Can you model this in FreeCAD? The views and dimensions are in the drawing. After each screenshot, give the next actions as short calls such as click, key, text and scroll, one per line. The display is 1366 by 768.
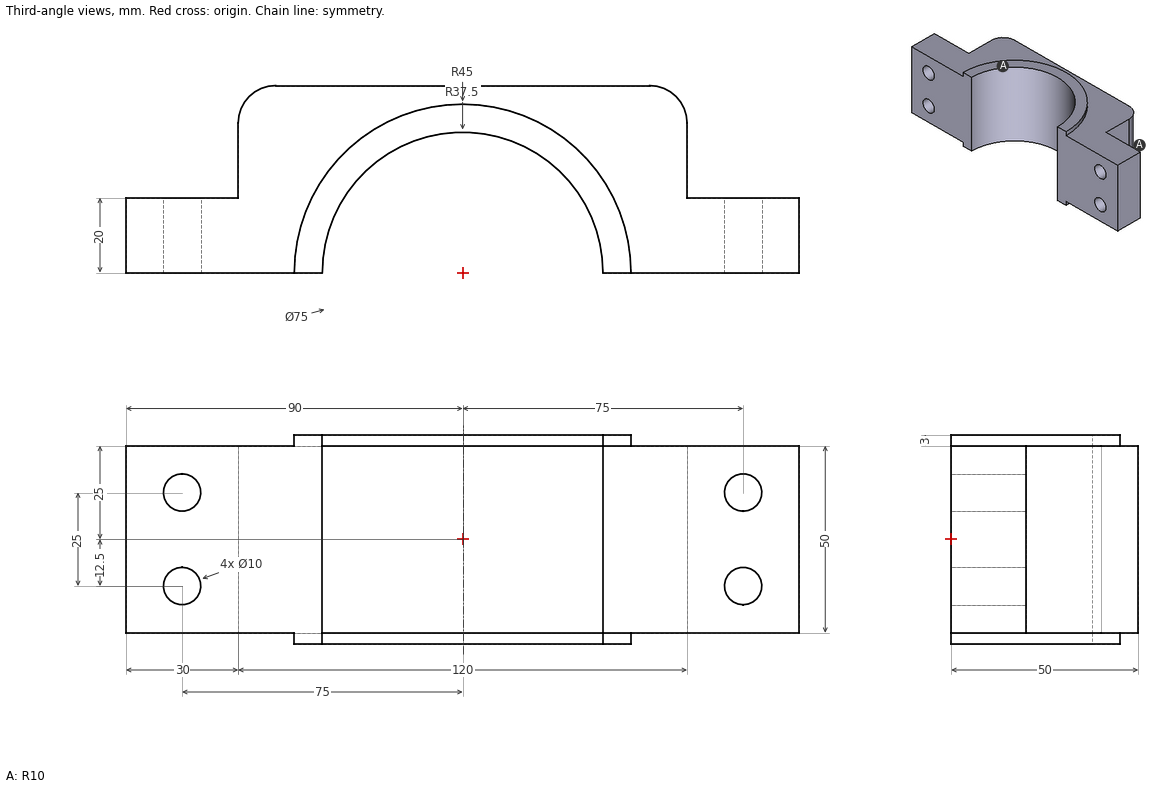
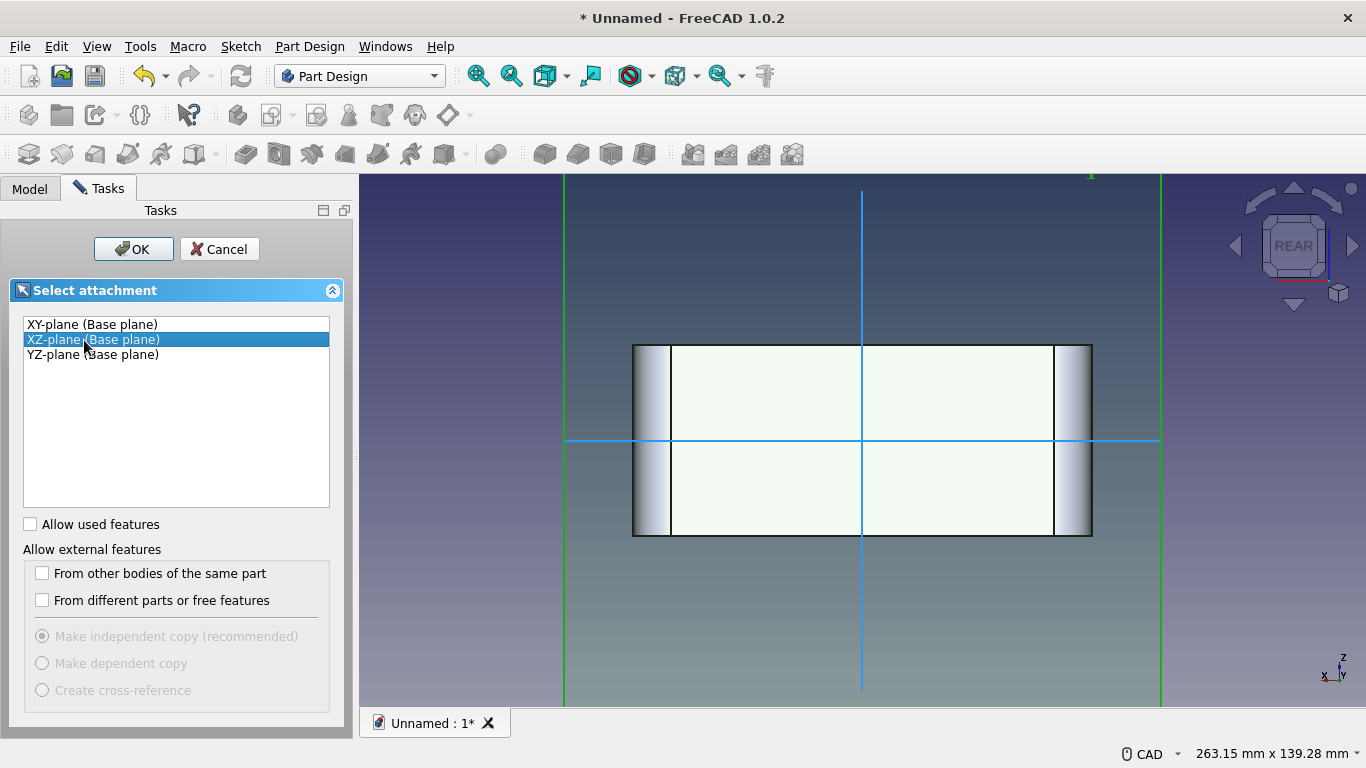
click(134, 249)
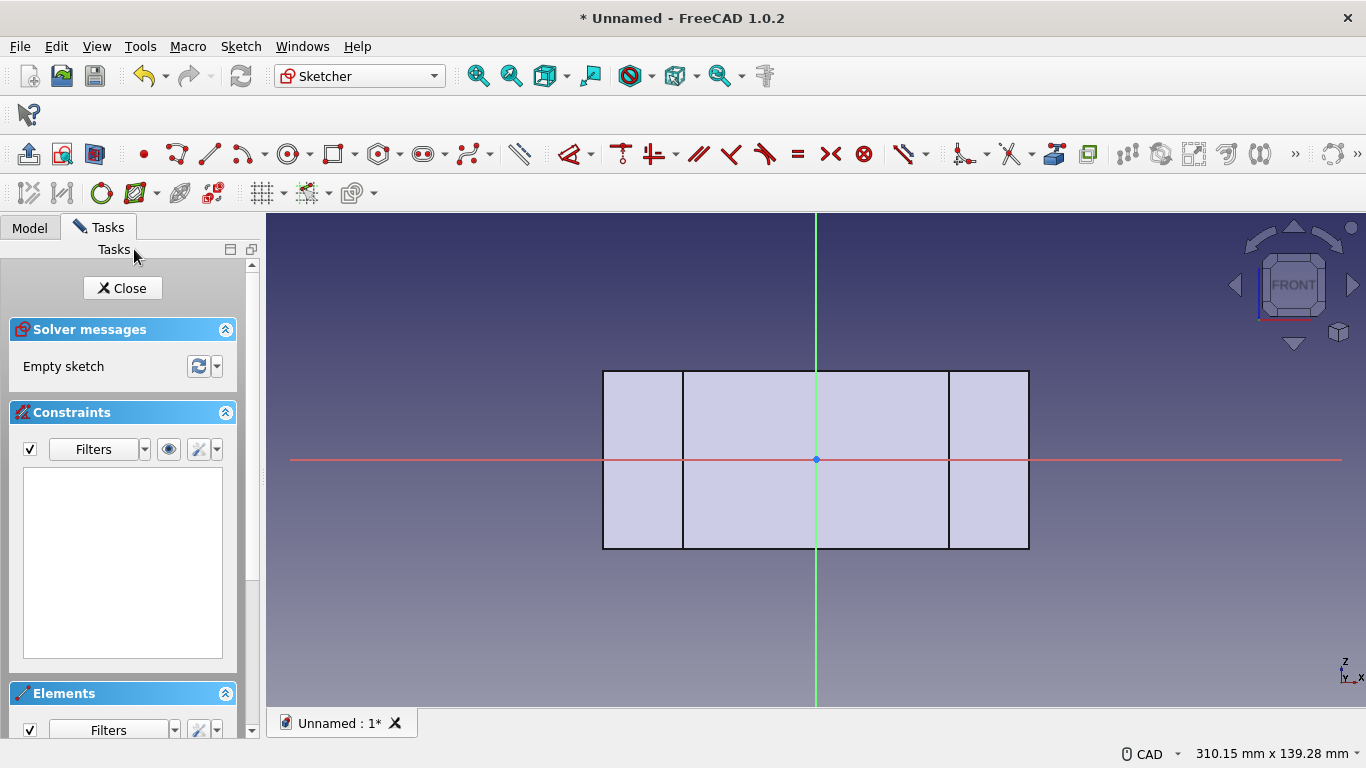
key(g)
key(r)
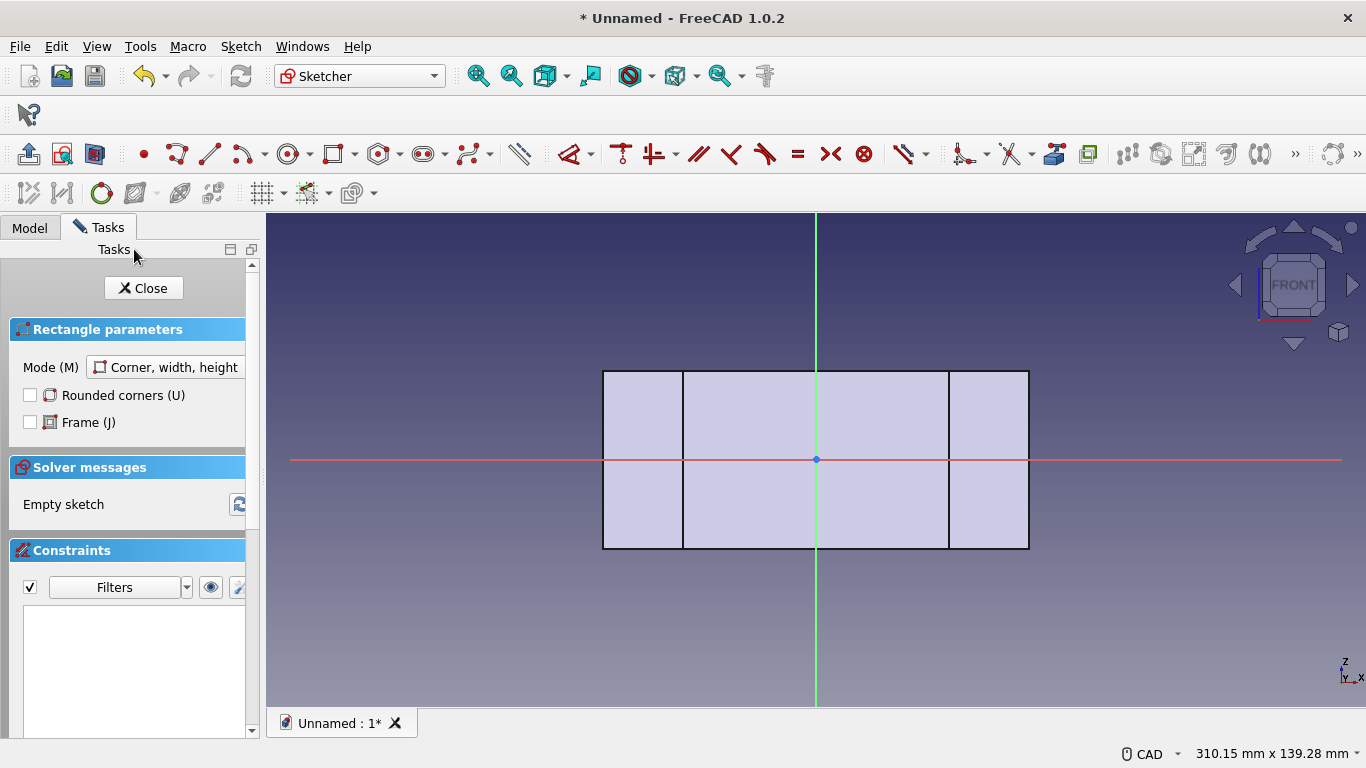
click(497, 371)
click(603, 549)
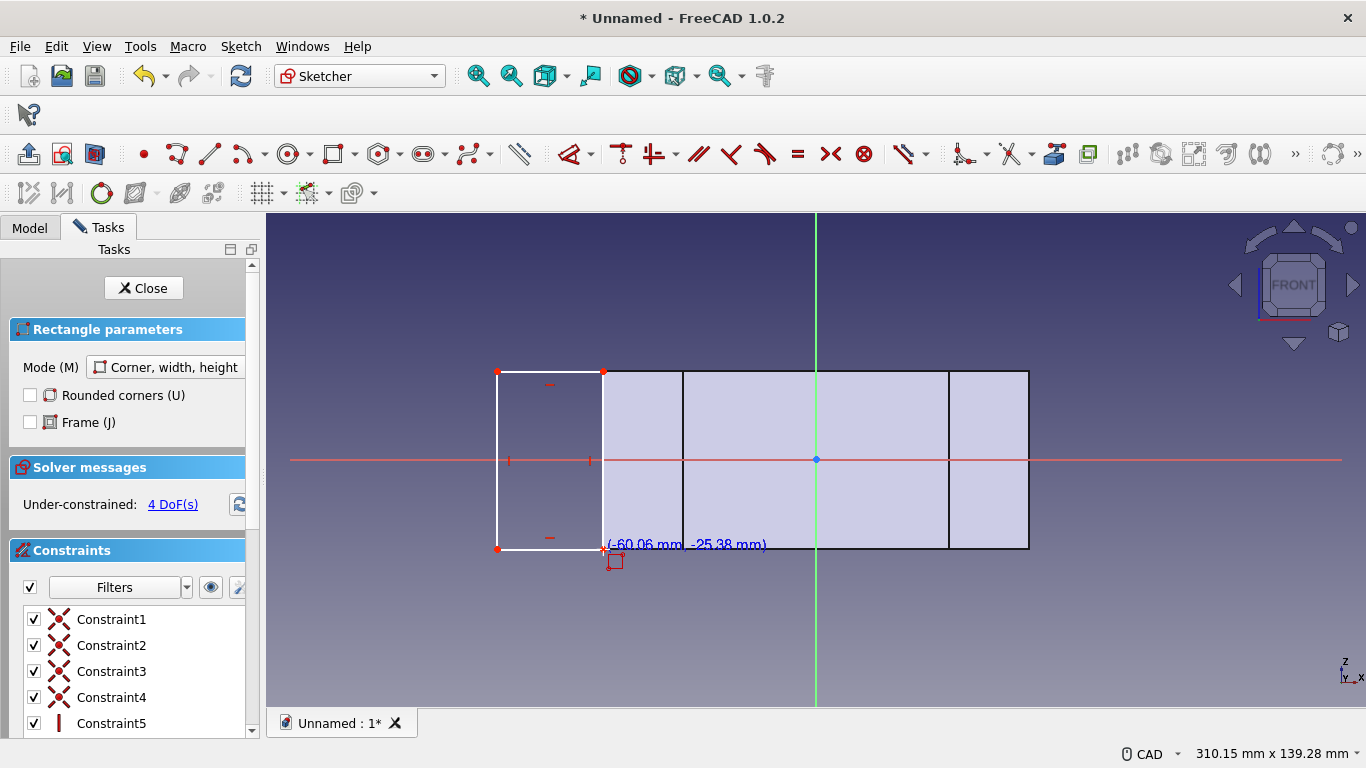
click(1029, 371)
click(1135, 549)
key(Escape)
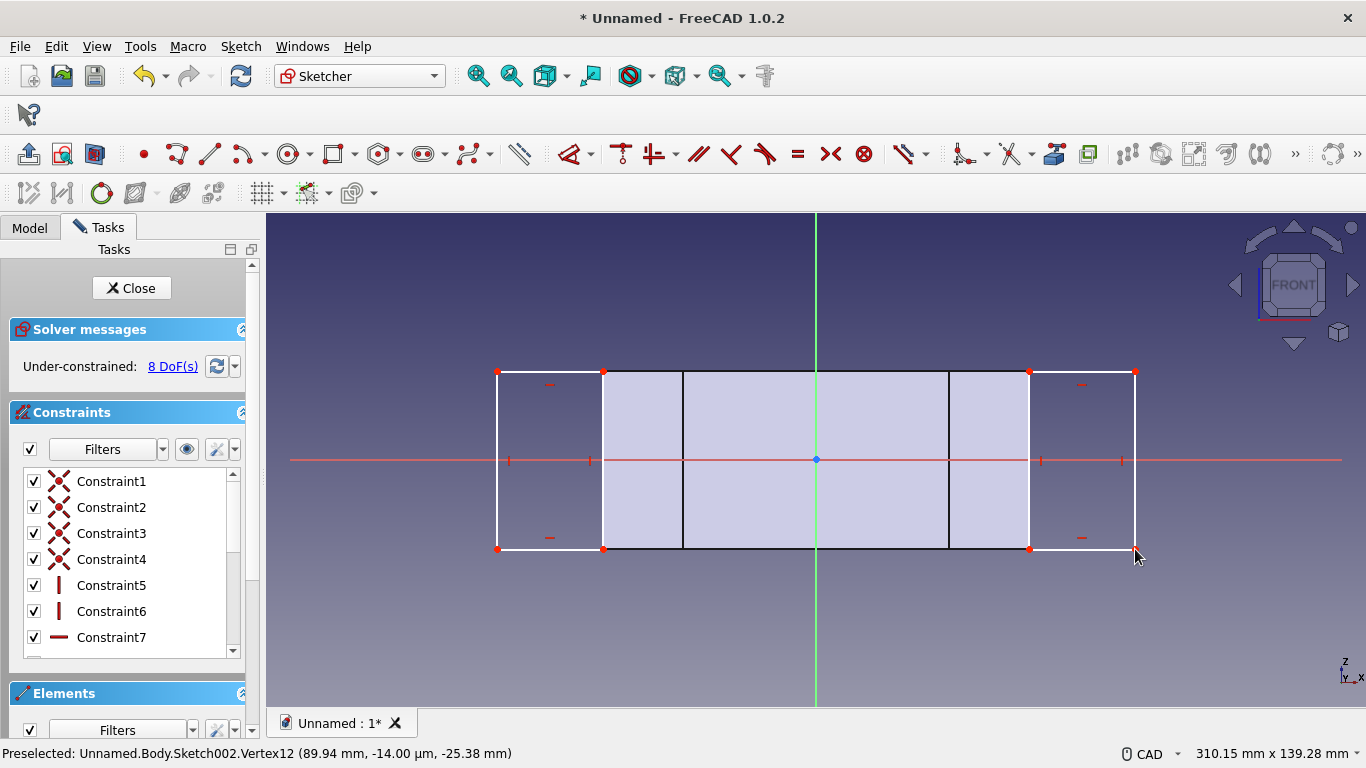
click(603, 372)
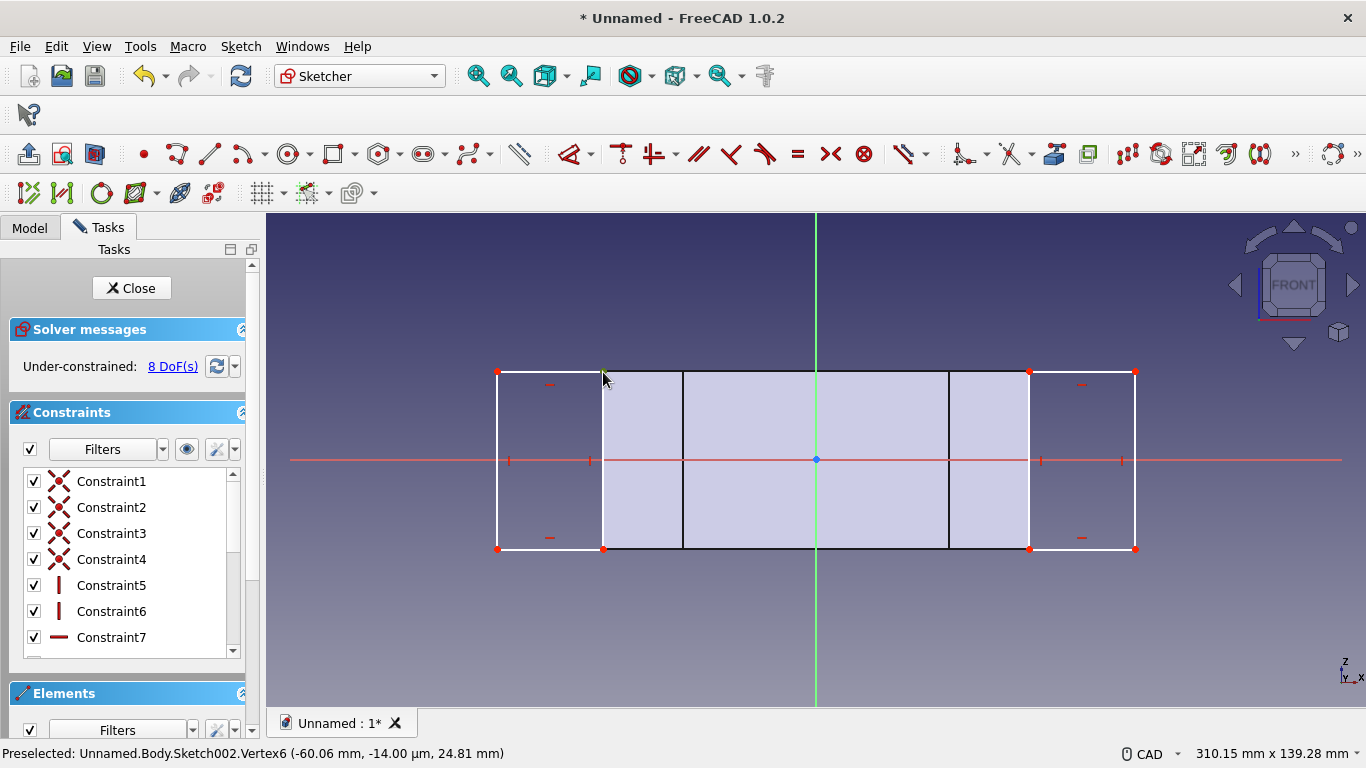
click(1029, 372)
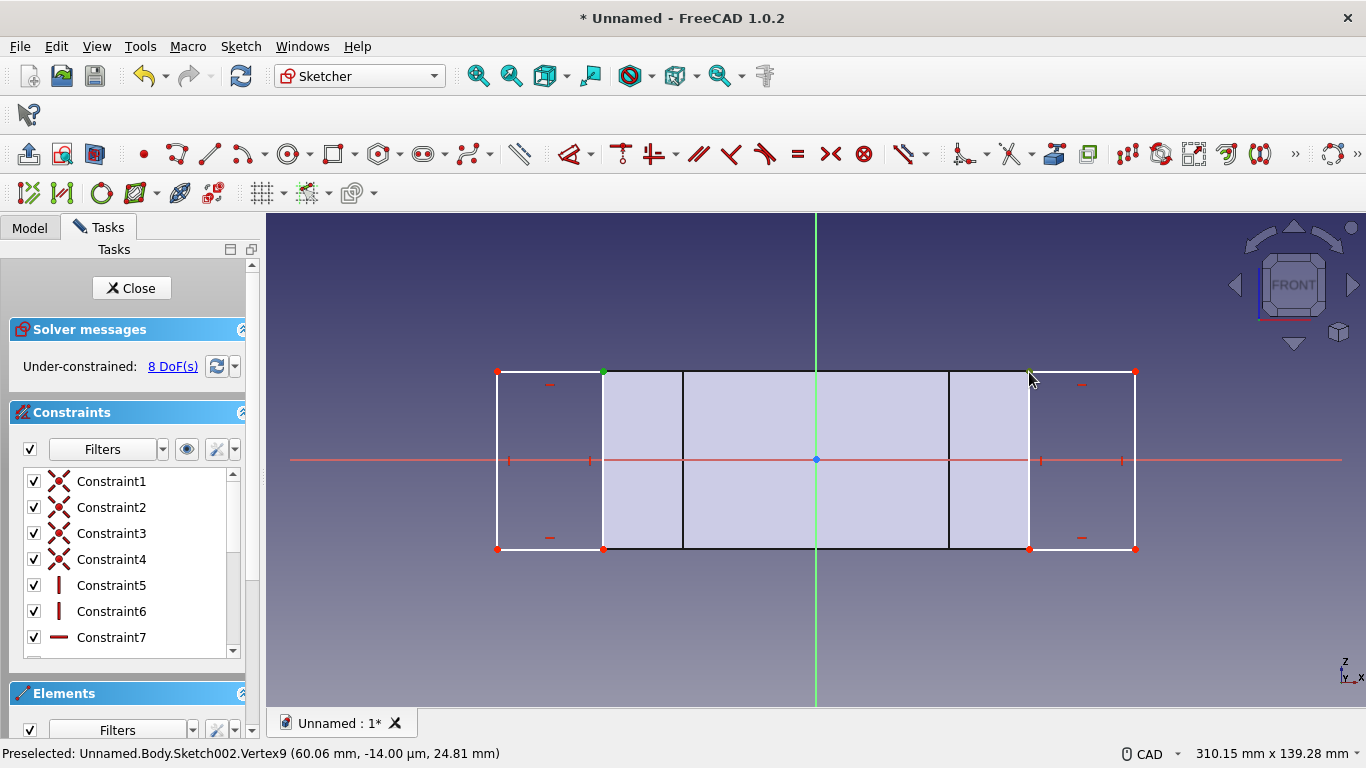
click(816, 648)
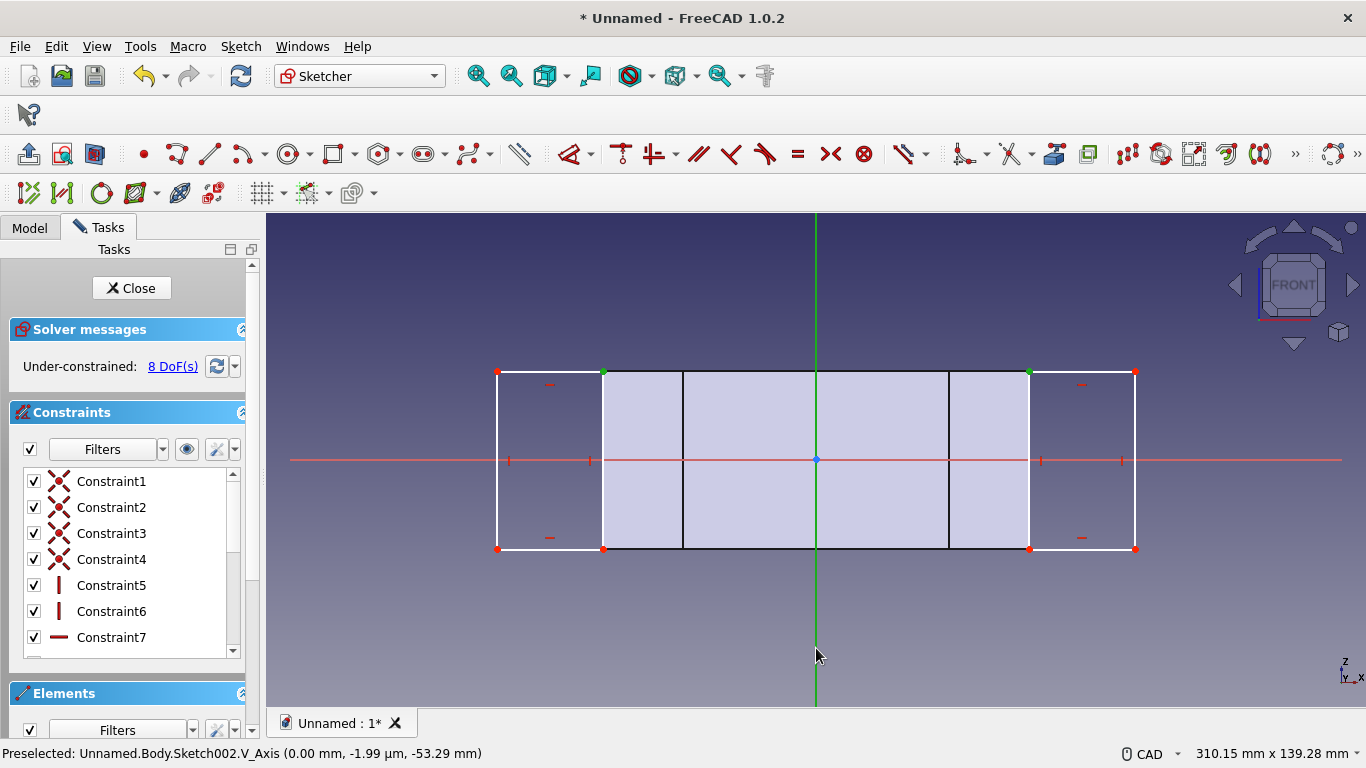
key(s)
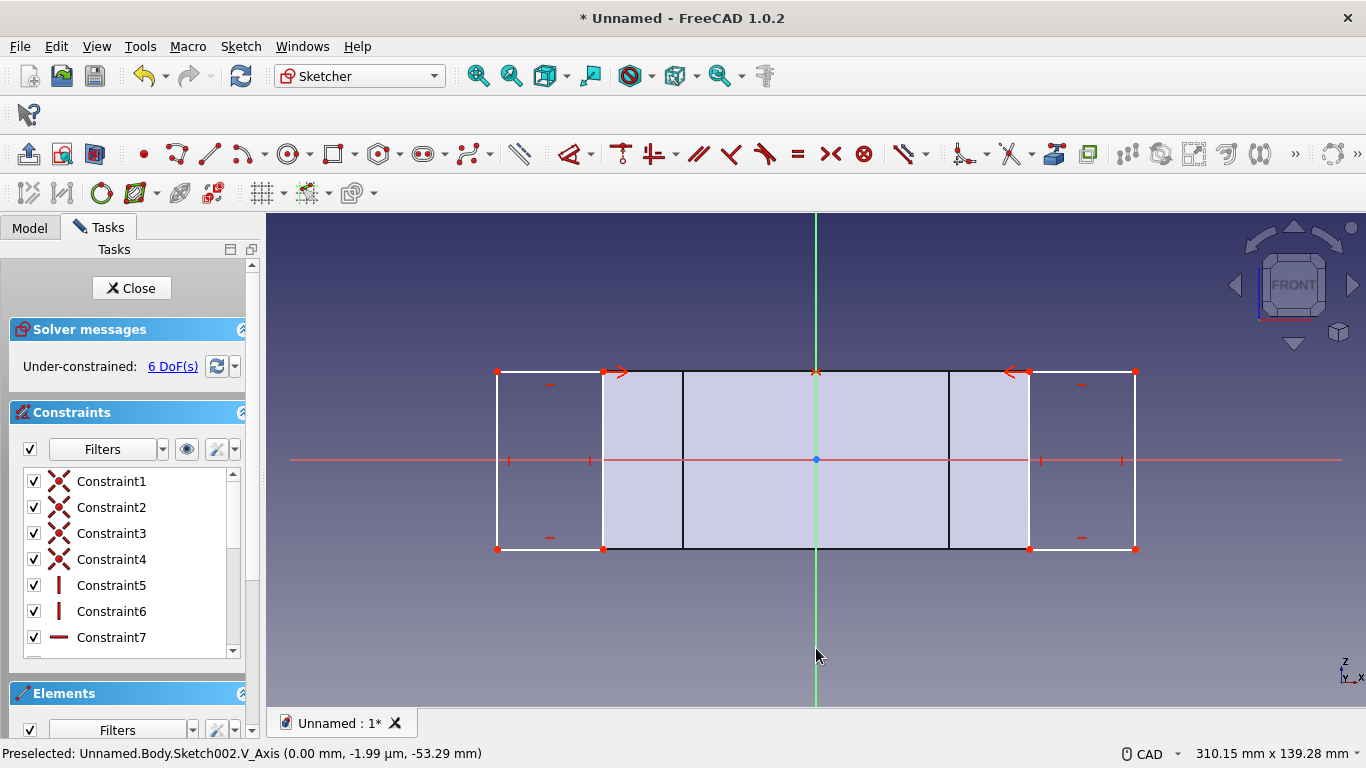
click(497, 550)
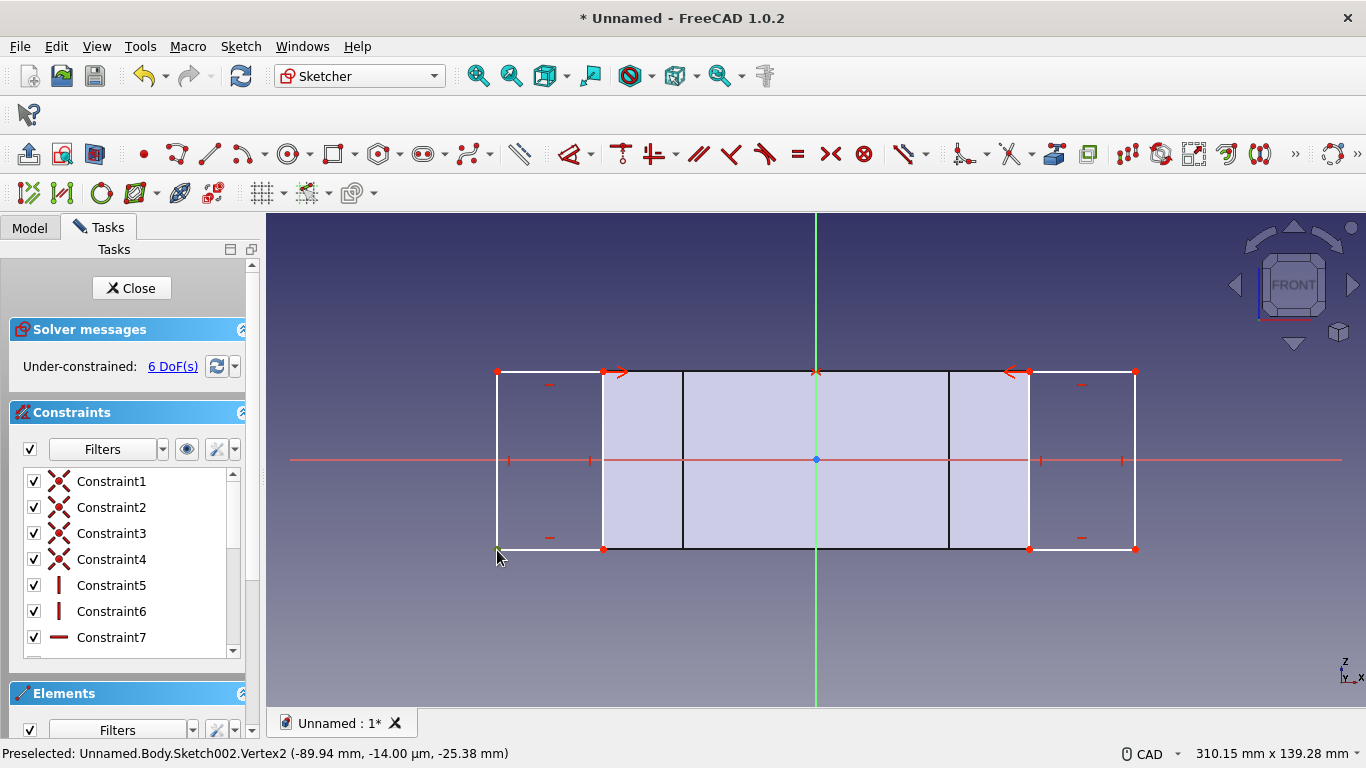
click(1135, 550)